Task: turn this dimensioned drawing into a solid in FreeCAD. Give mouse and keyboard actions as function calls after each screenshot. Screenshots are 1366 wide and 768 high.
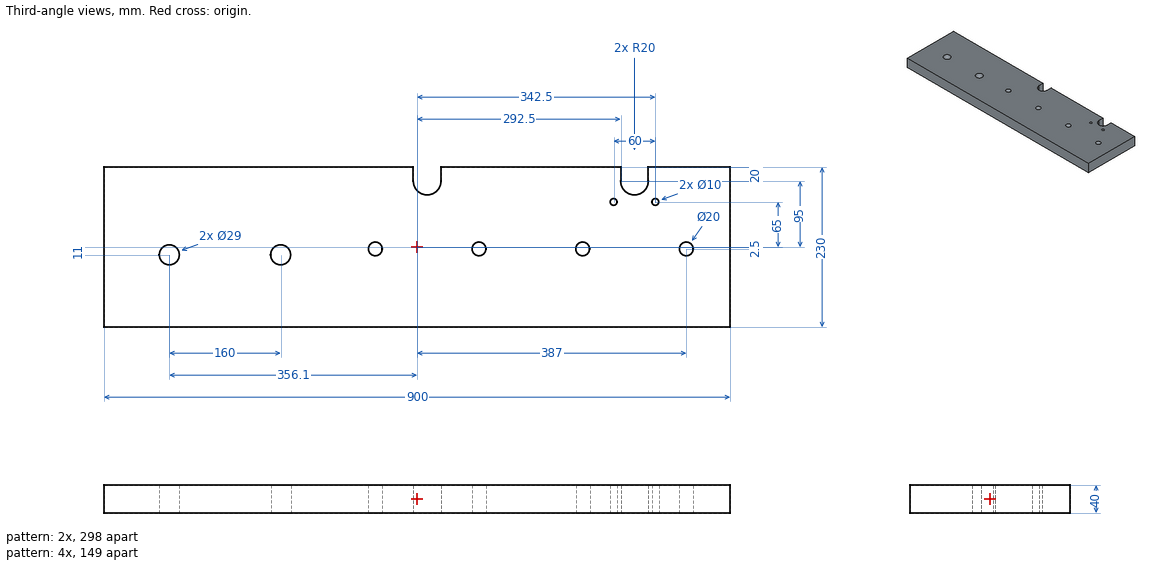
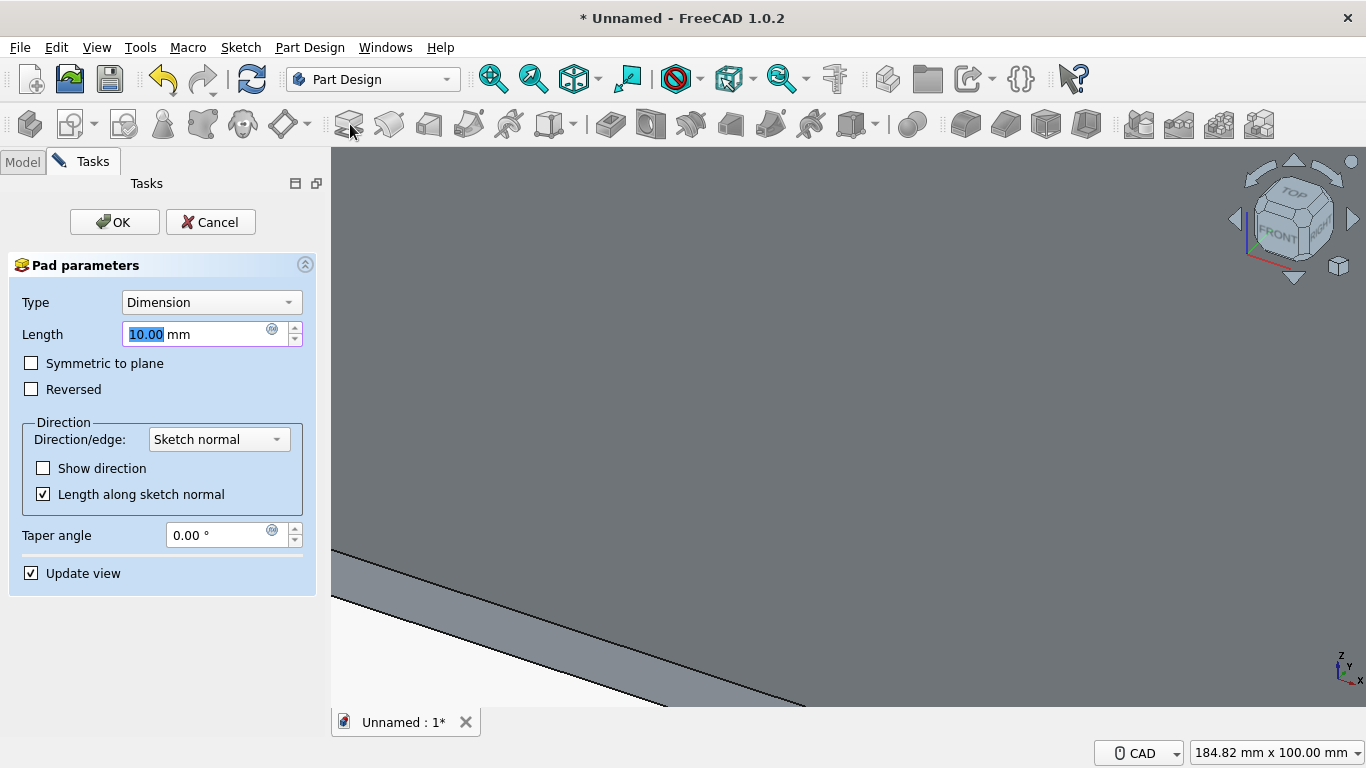
text(40)
key(Tab)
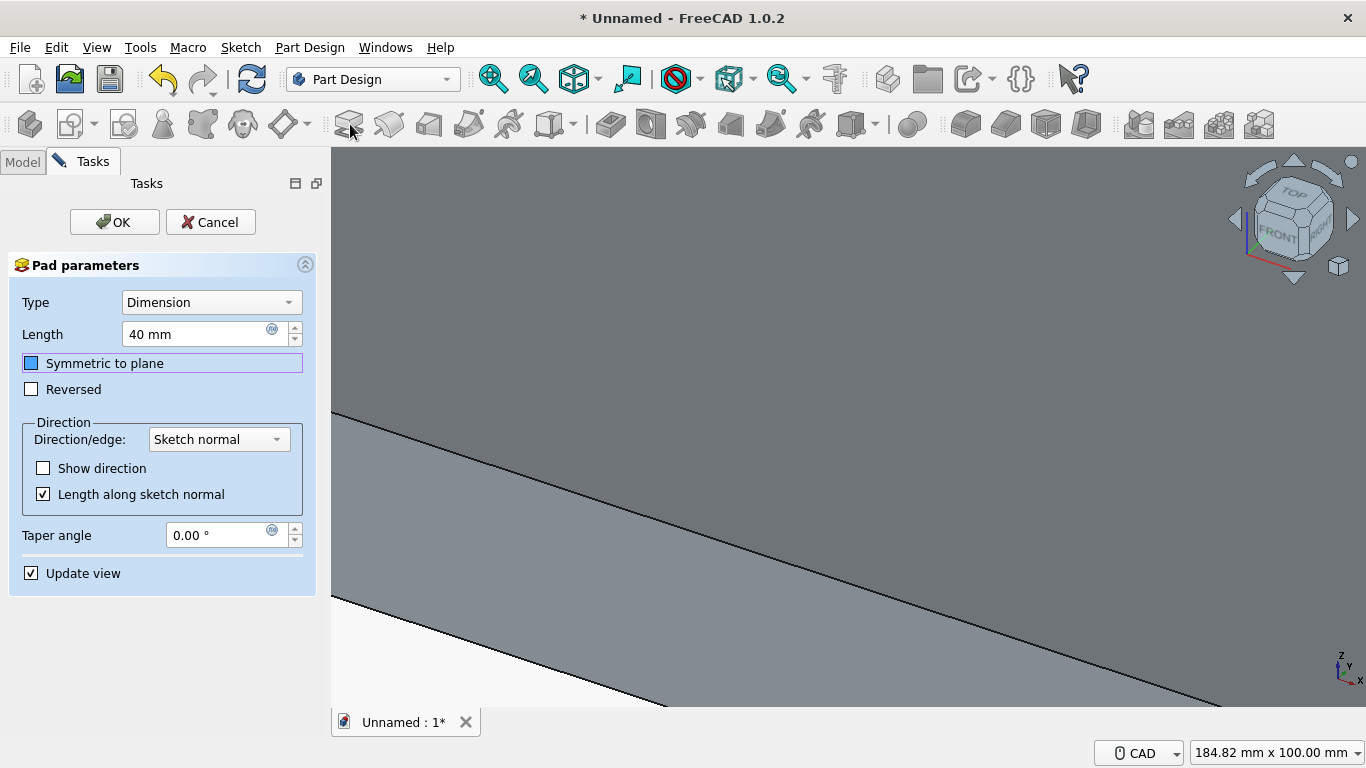
click(30, 363)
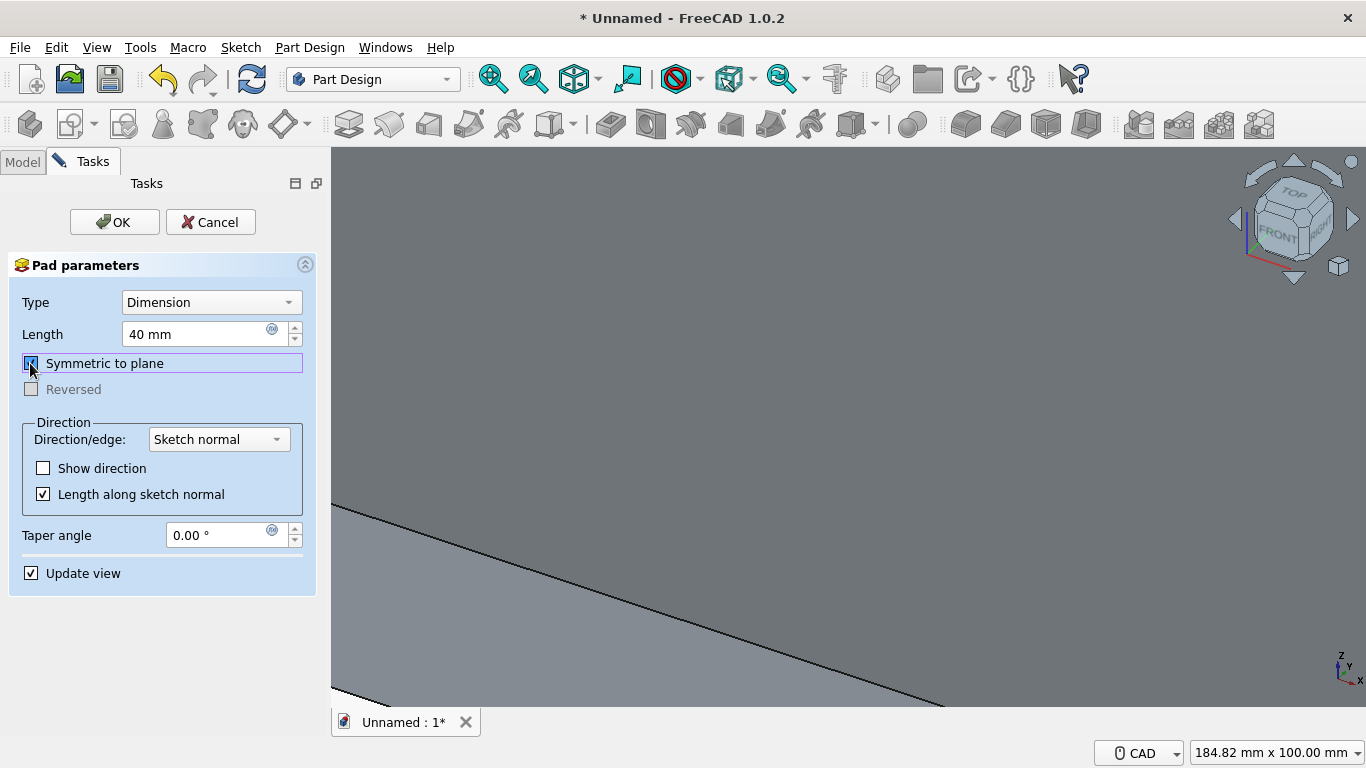
click(115, 222)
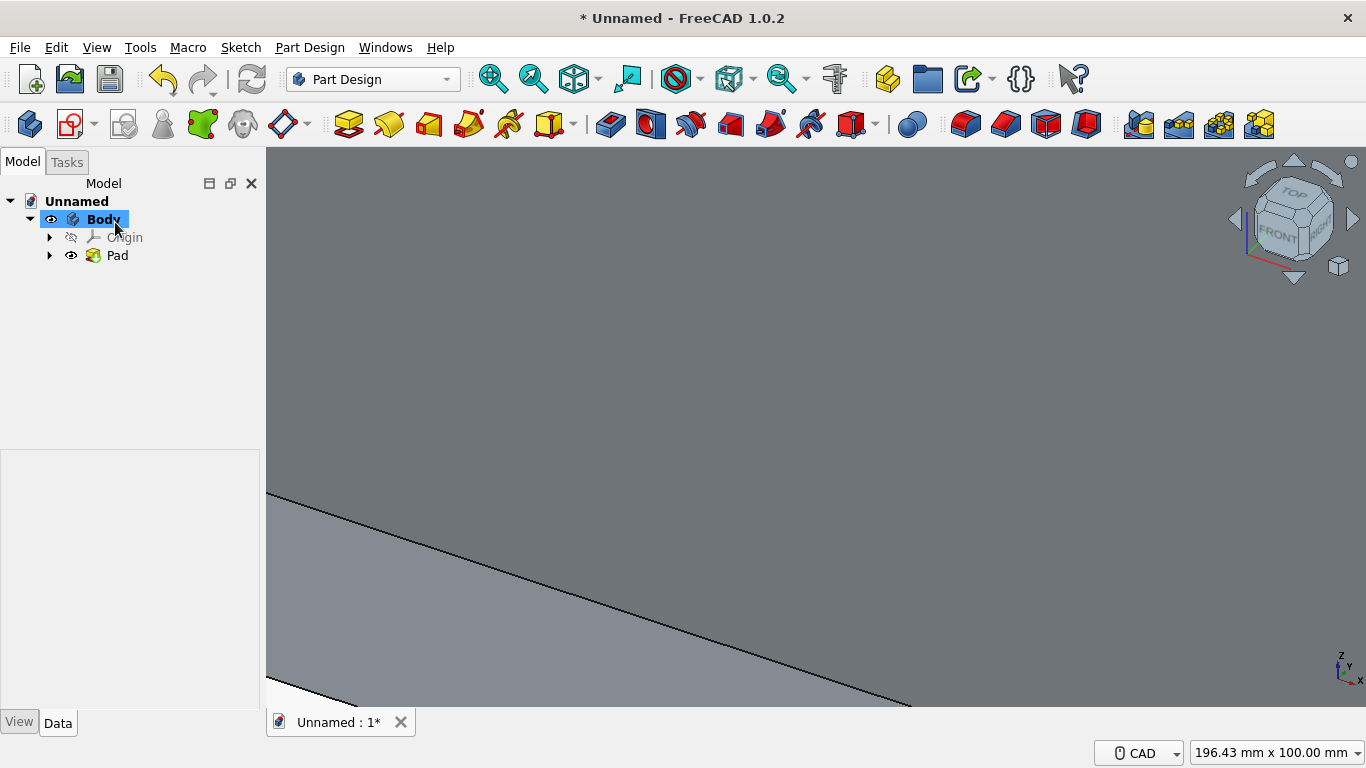
key(v)
key(f)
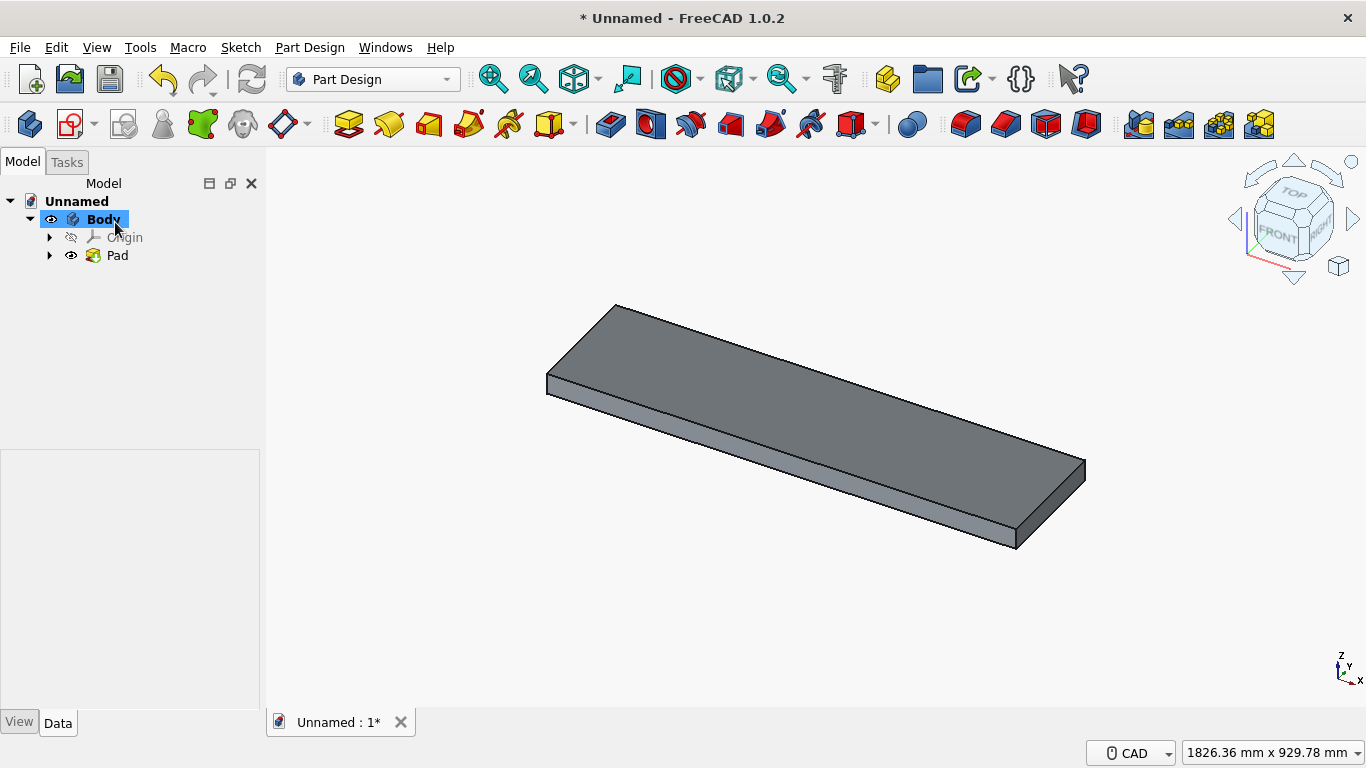
click(950, 461)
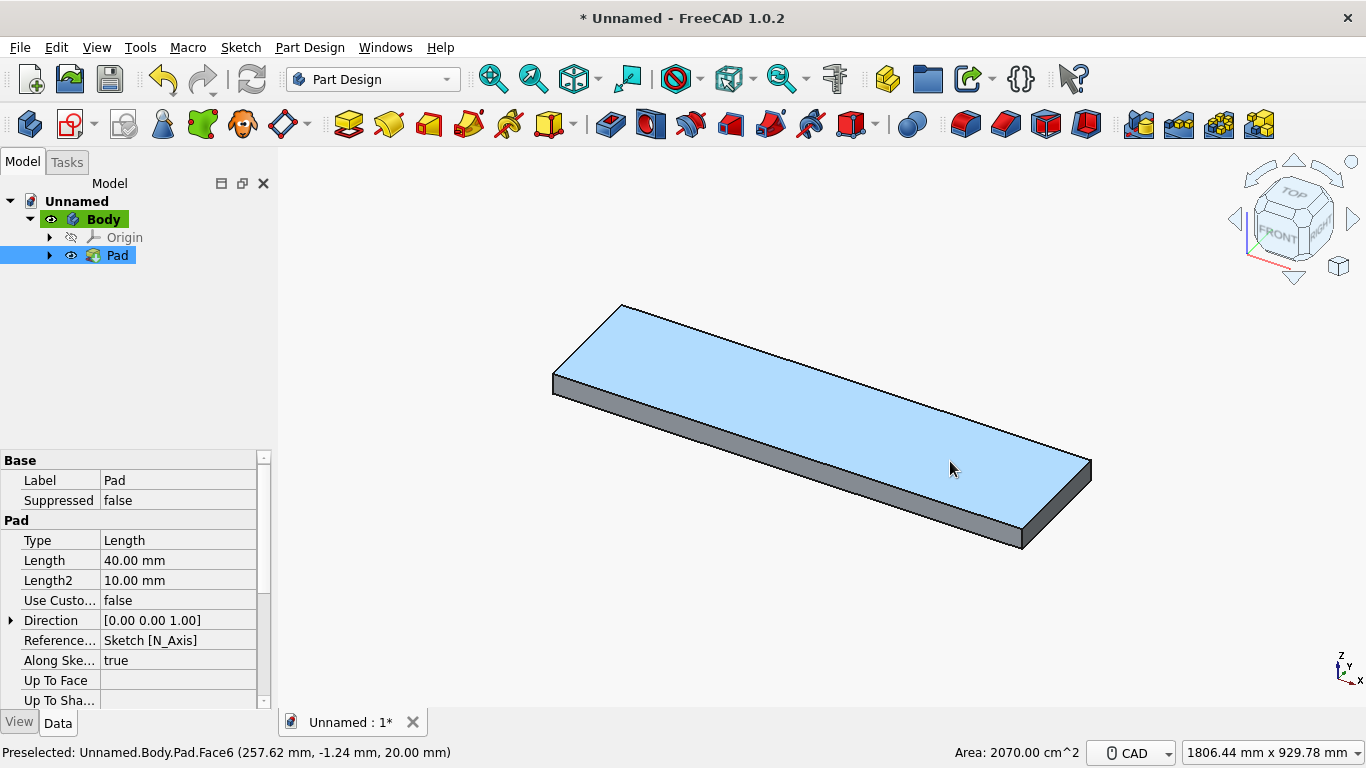
click(70, 124)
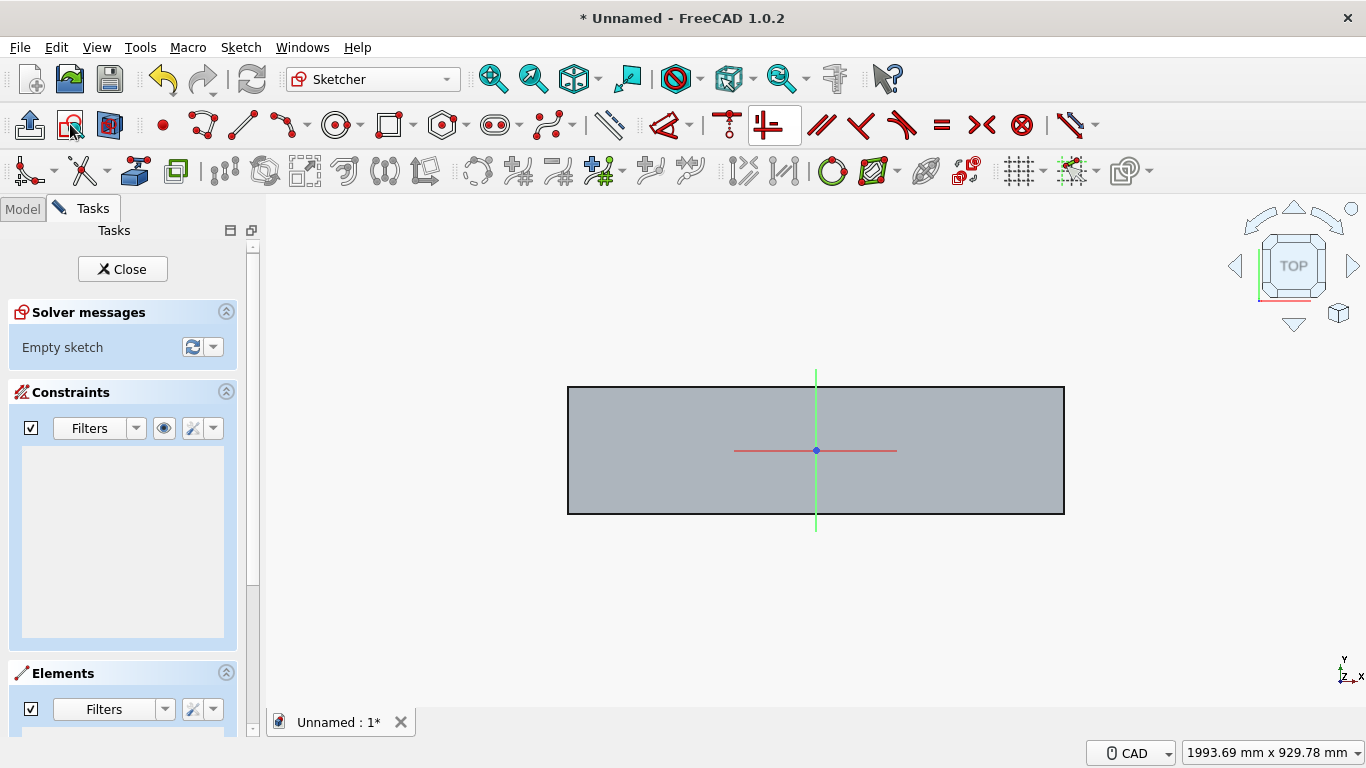
scroll(1044, 452, up, 15)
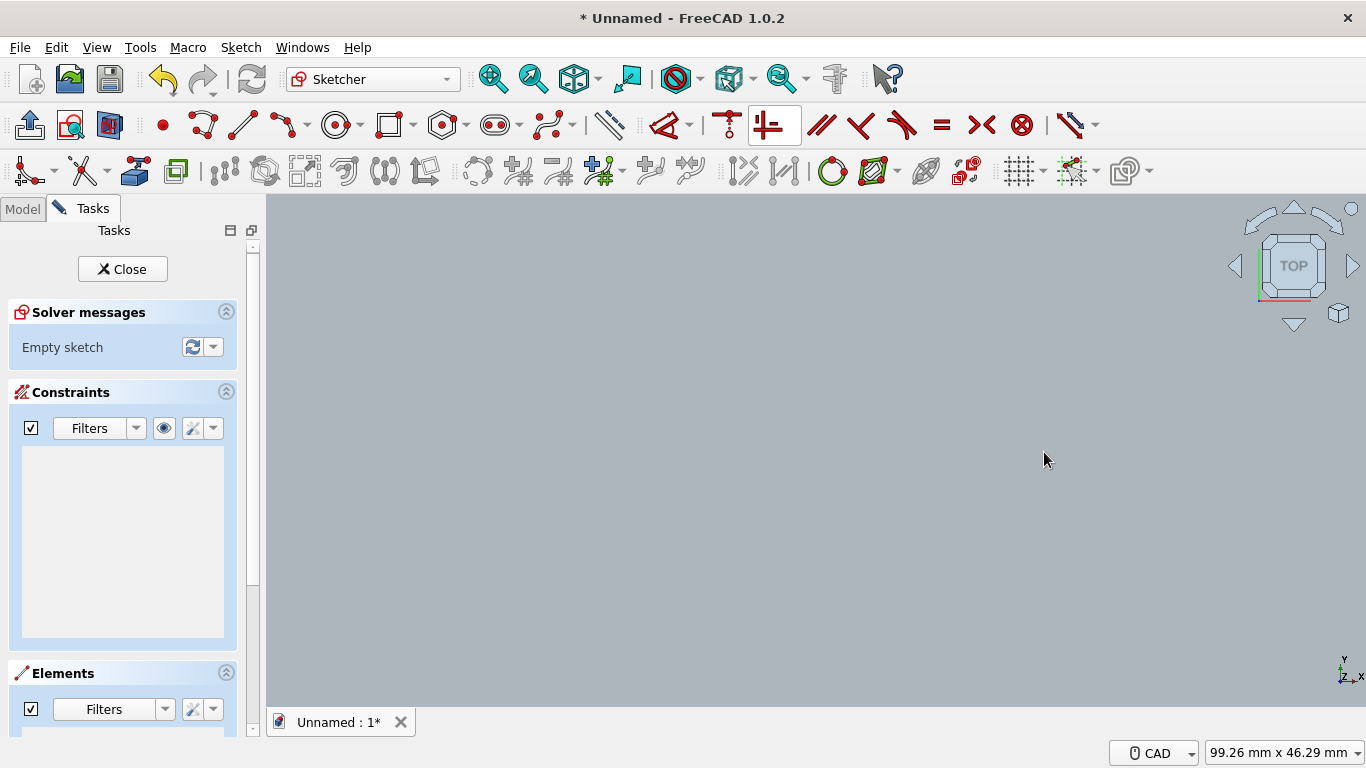
scroll(724, 419, up, 2)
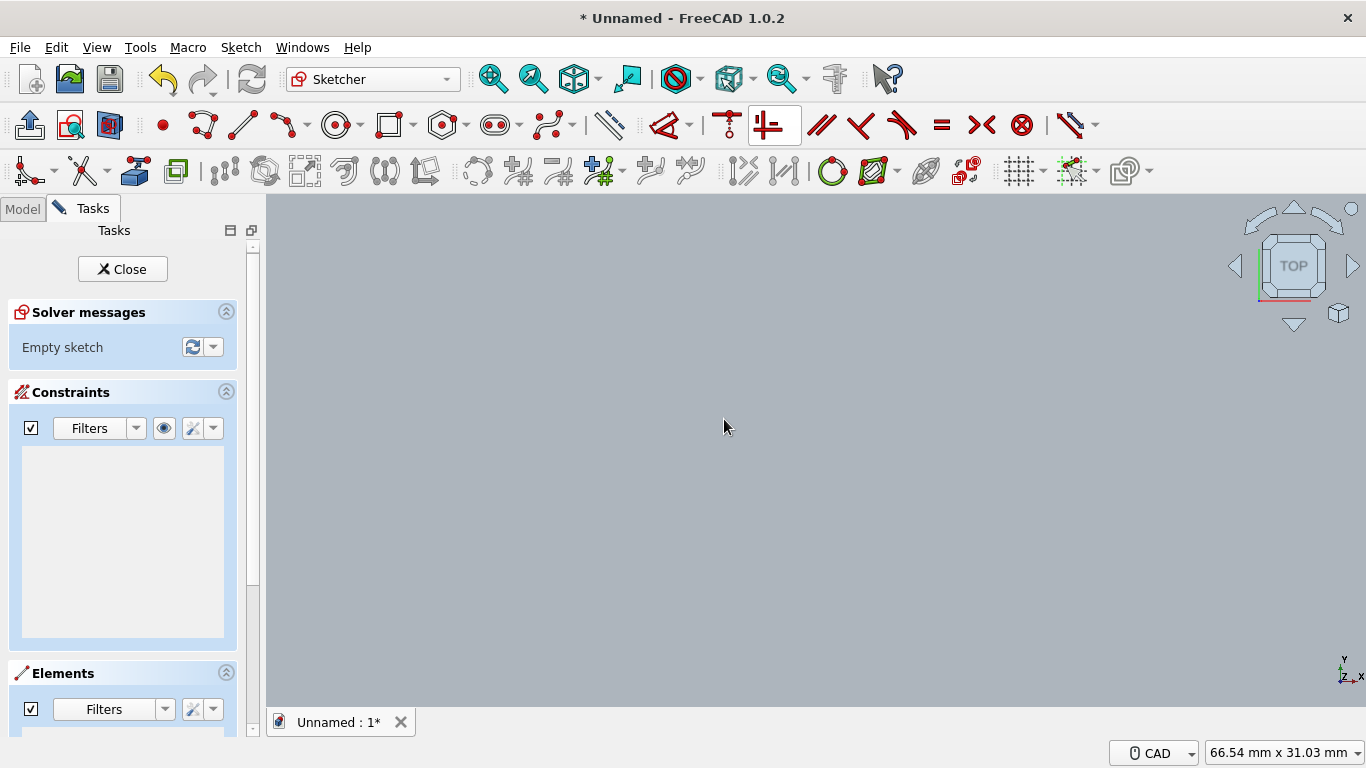
key(g)
key(c)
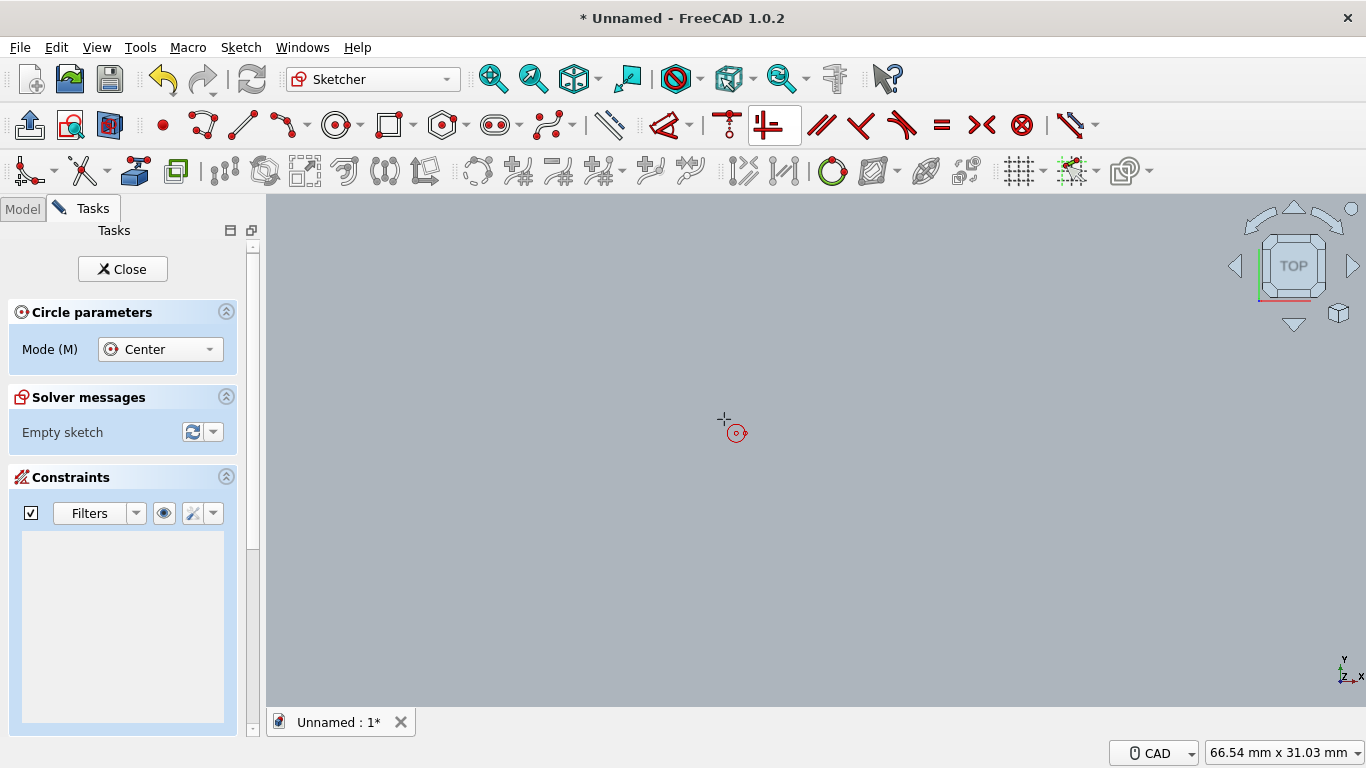
click(747, 450)
move(864, 333)